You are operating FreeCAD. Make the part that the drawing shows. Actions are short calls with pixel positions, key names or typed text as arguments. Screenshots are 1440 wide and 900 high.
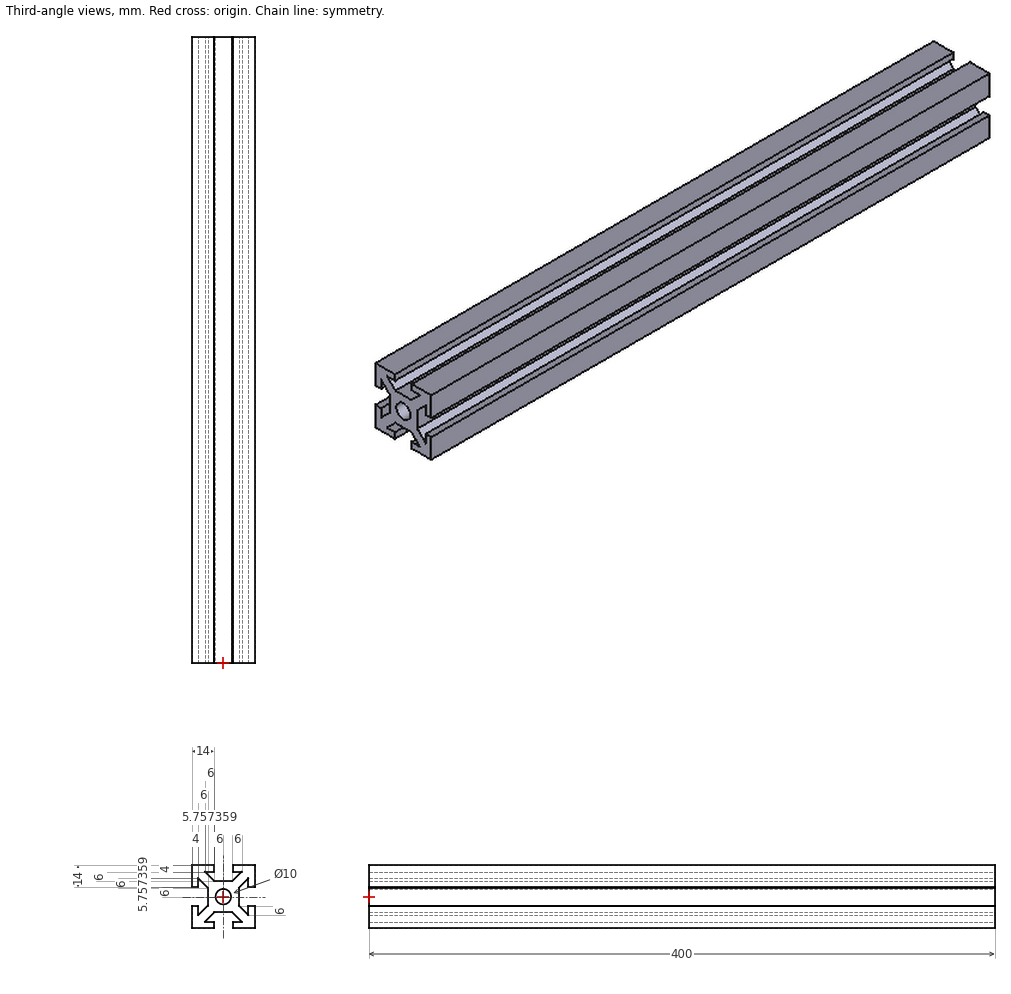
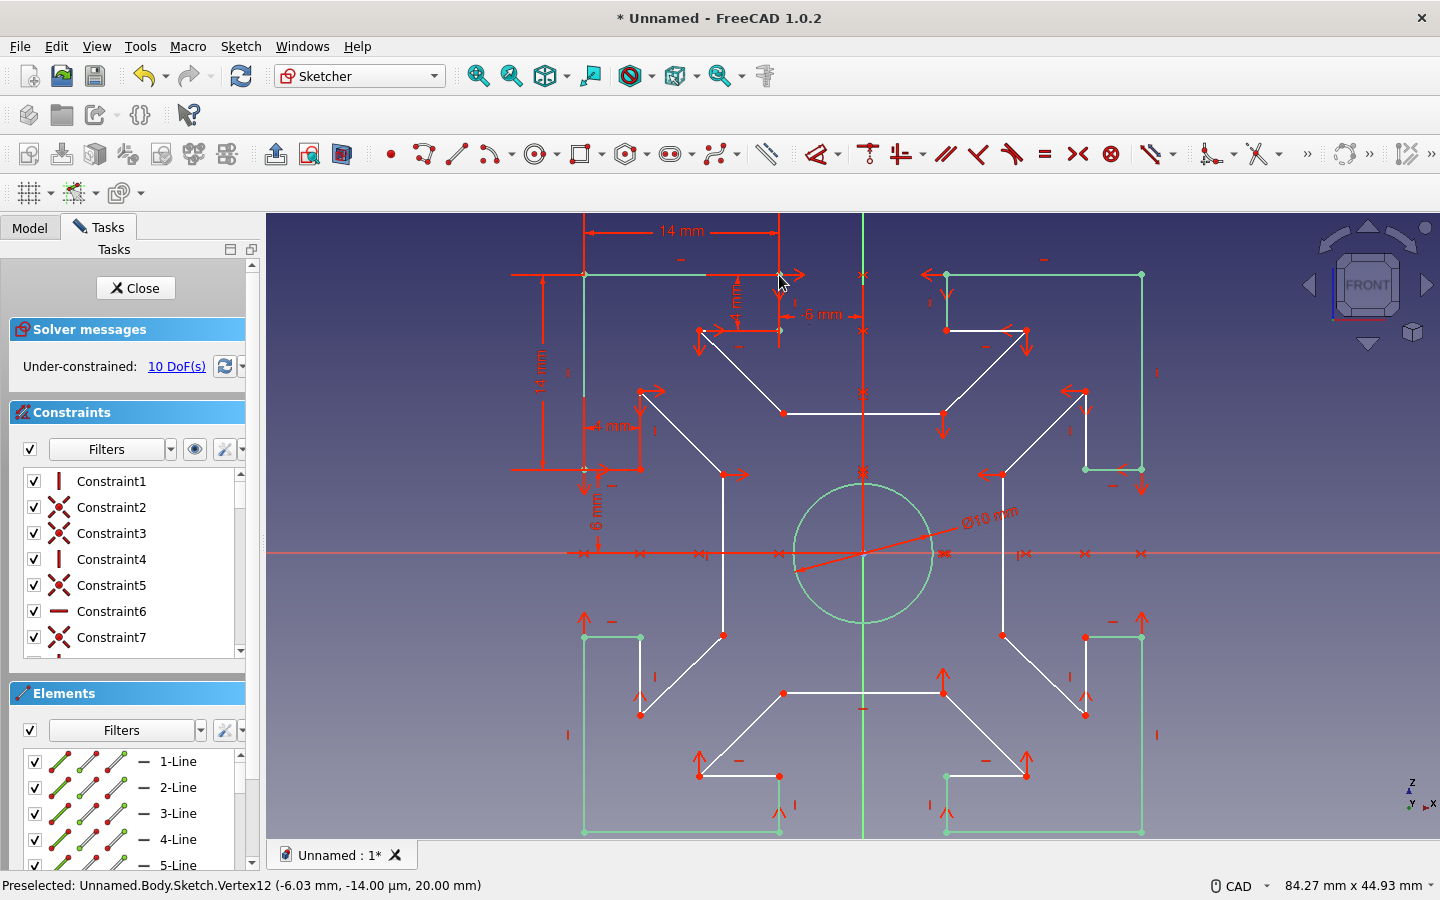
click(698, 450)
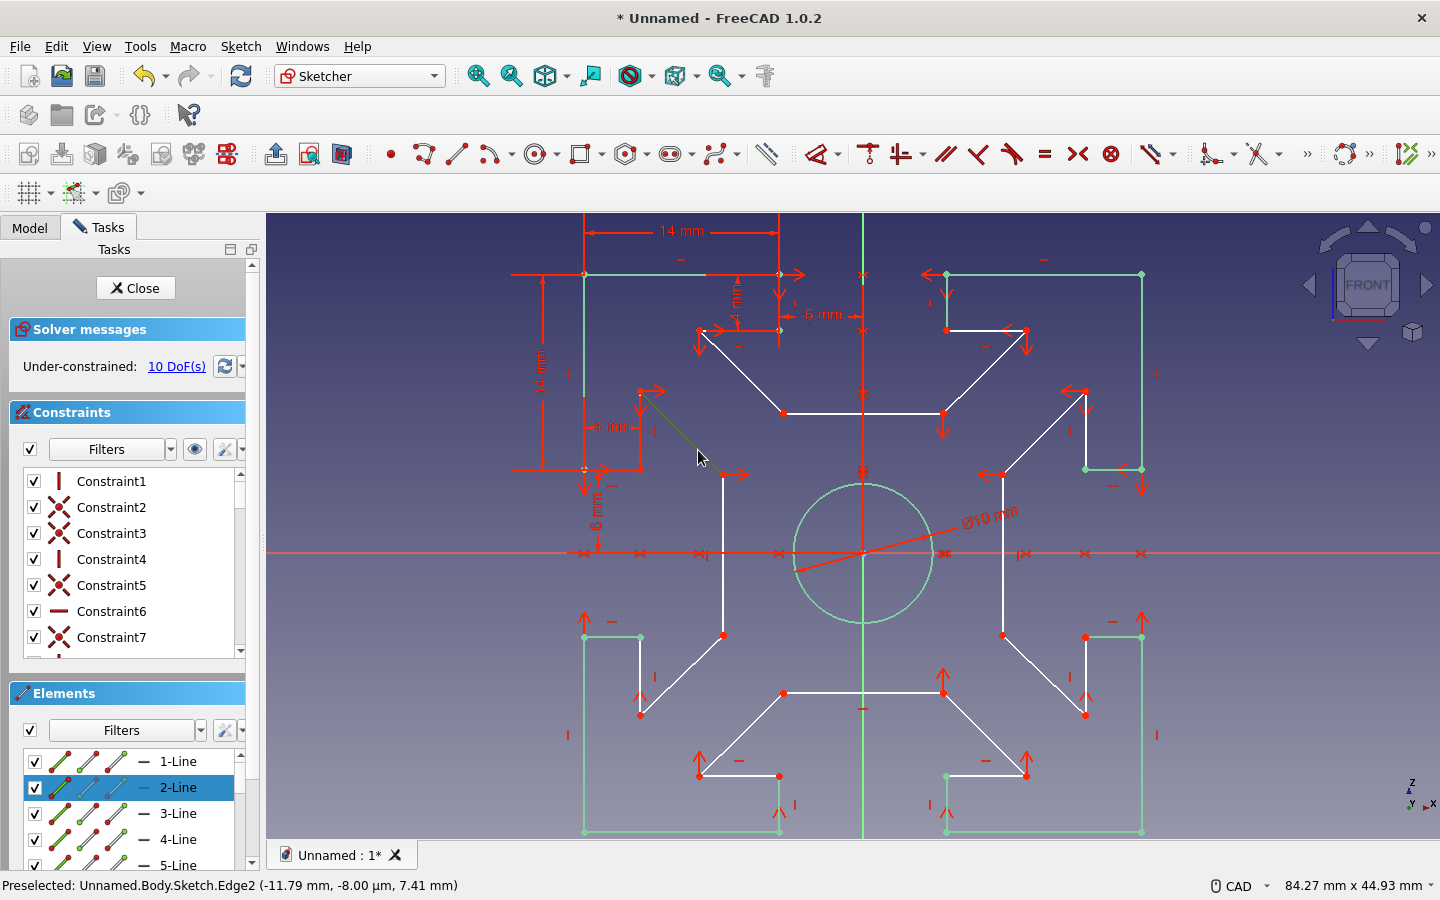
click(838, 154)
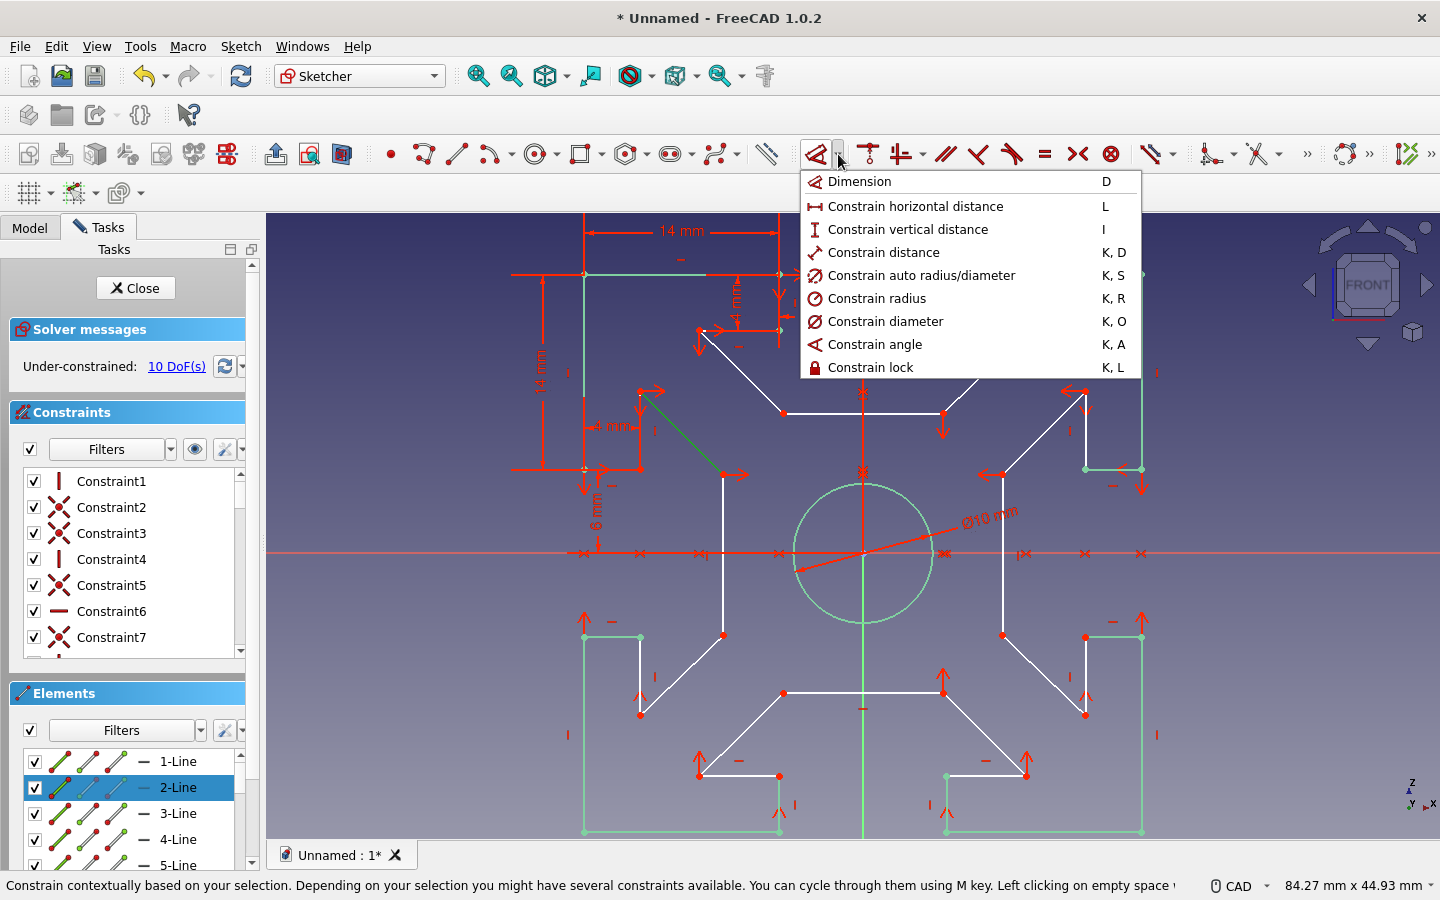
click(971, 206)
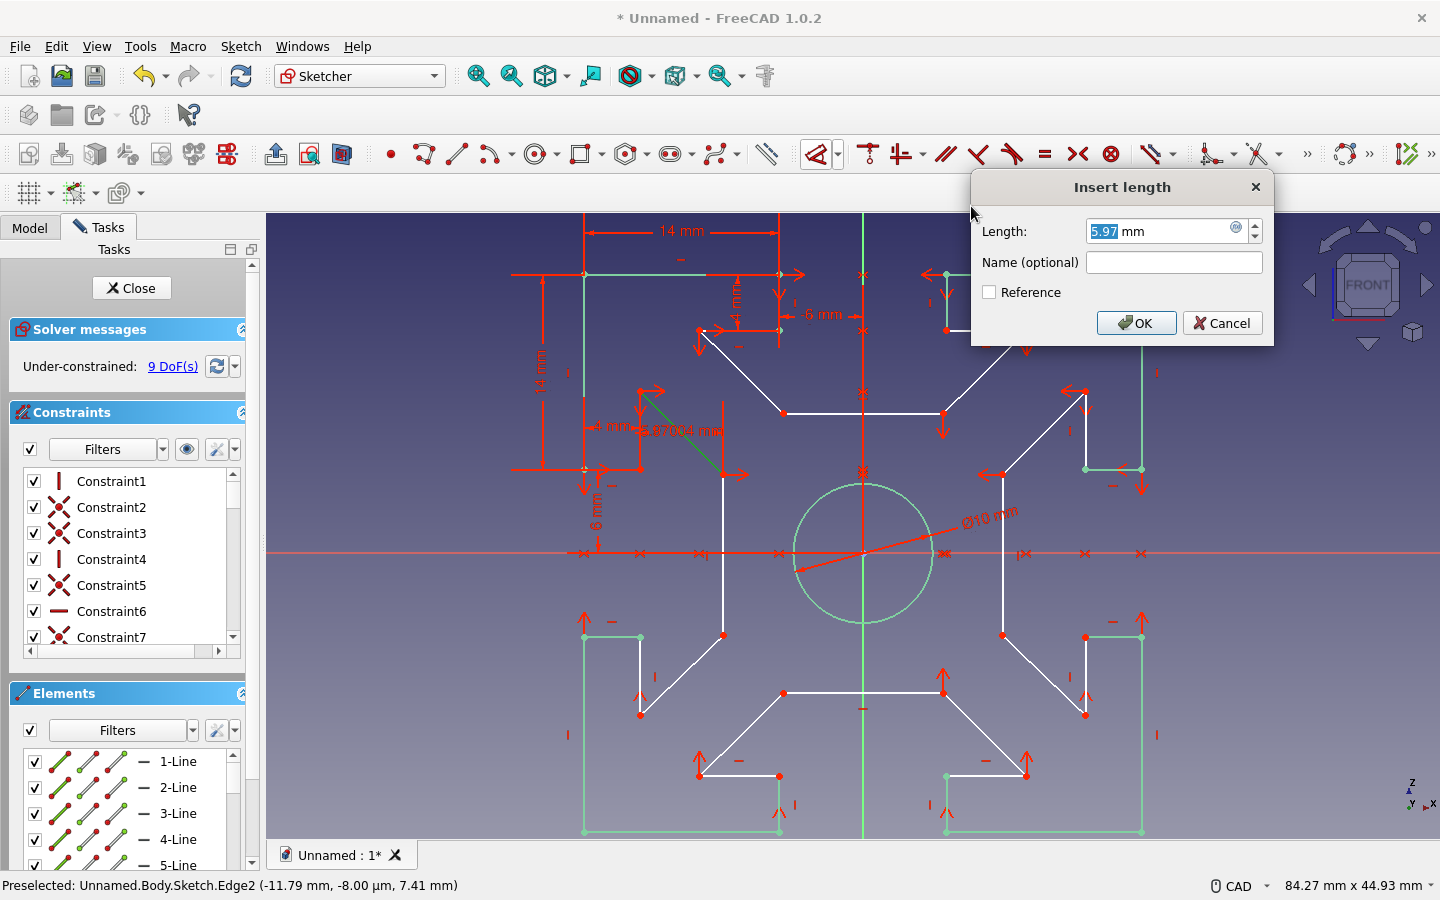
text(6)
key(Return)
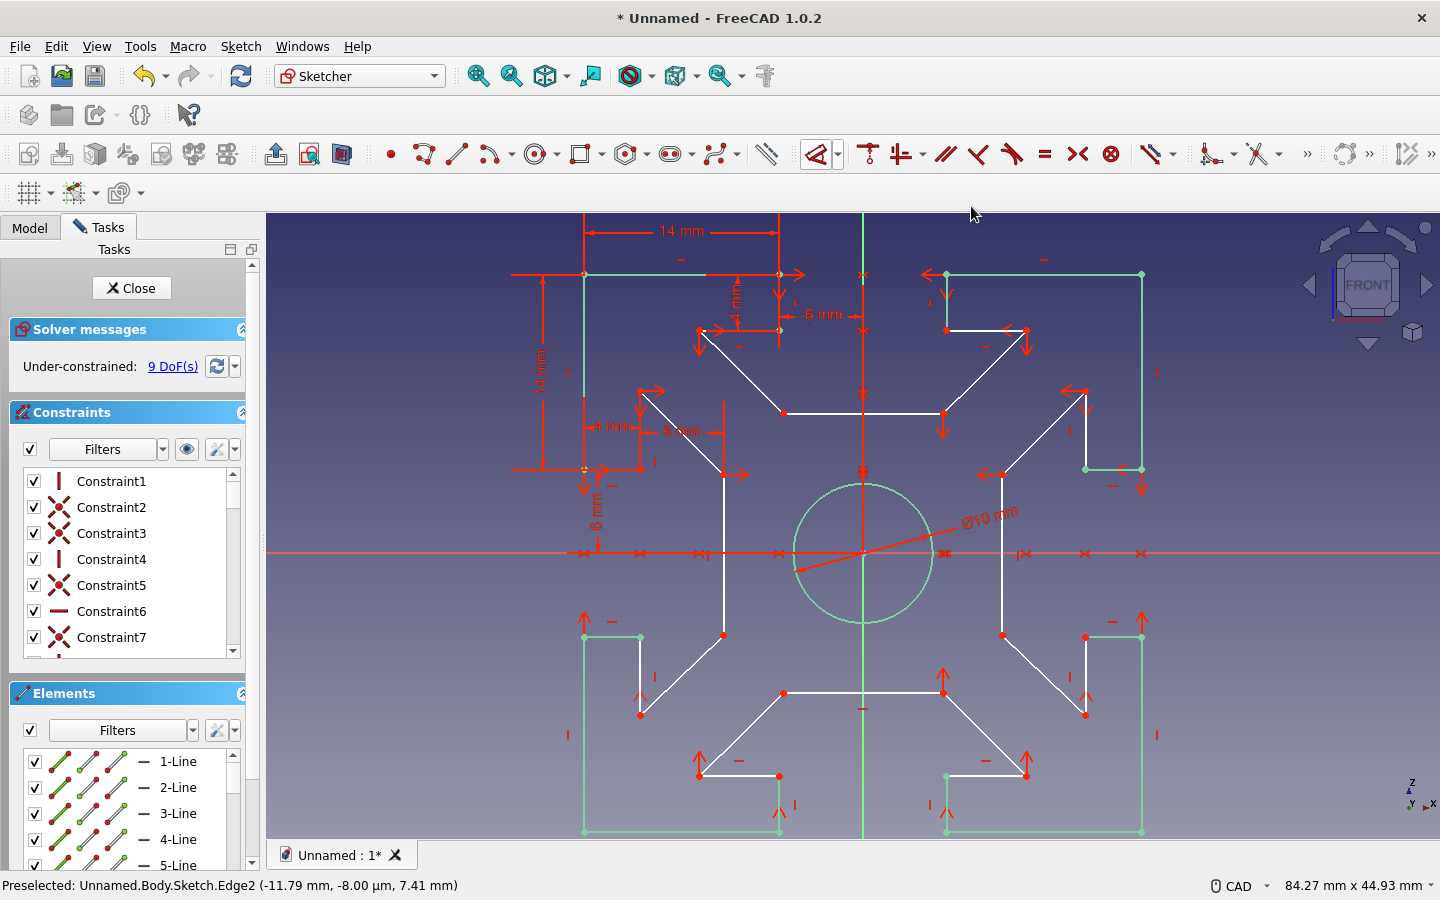
click(699, 450)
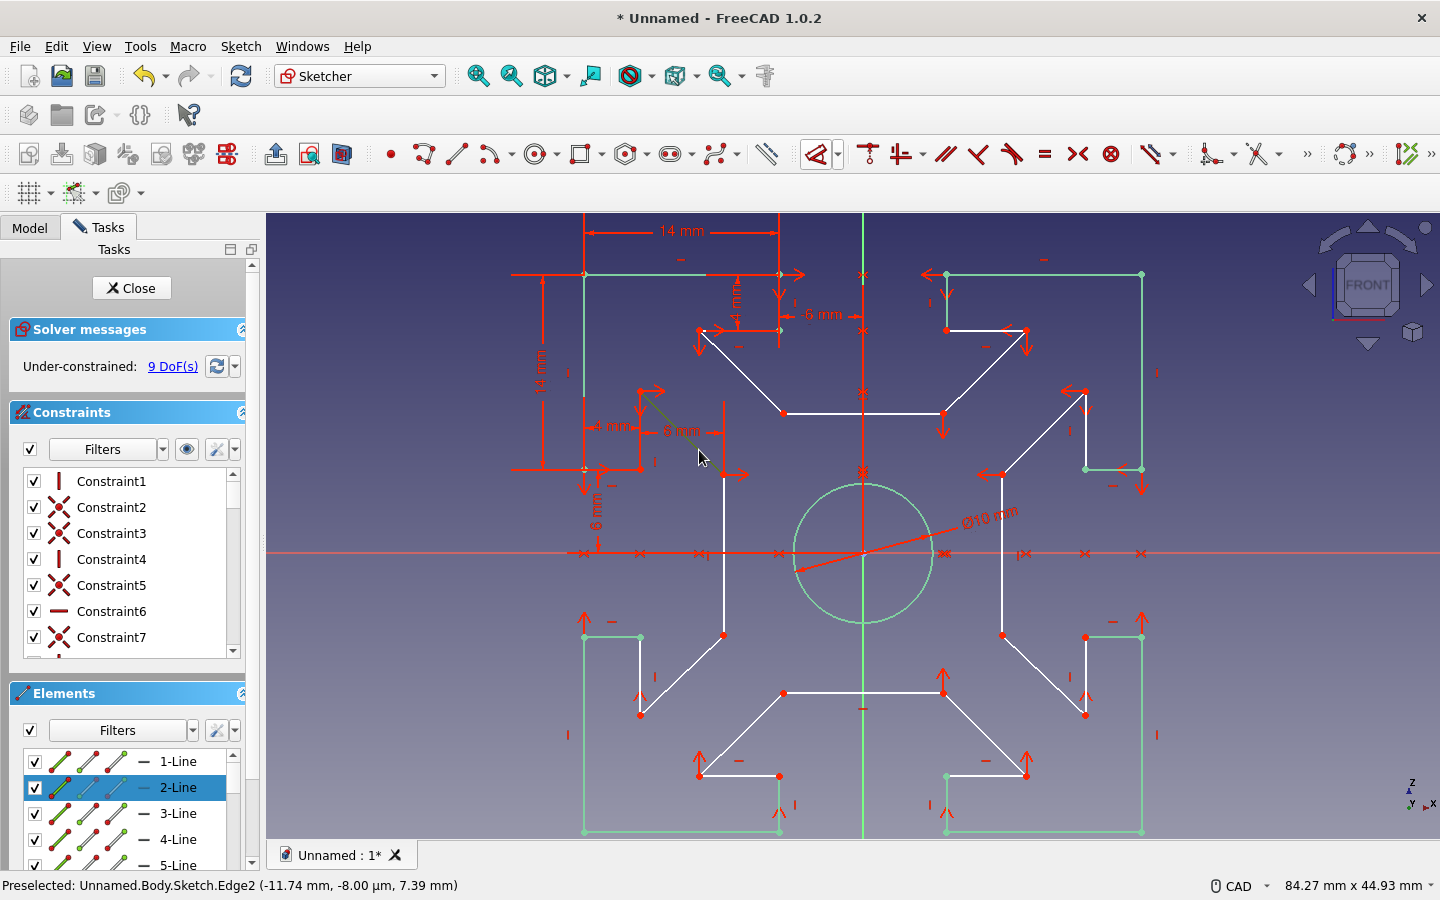
key(i)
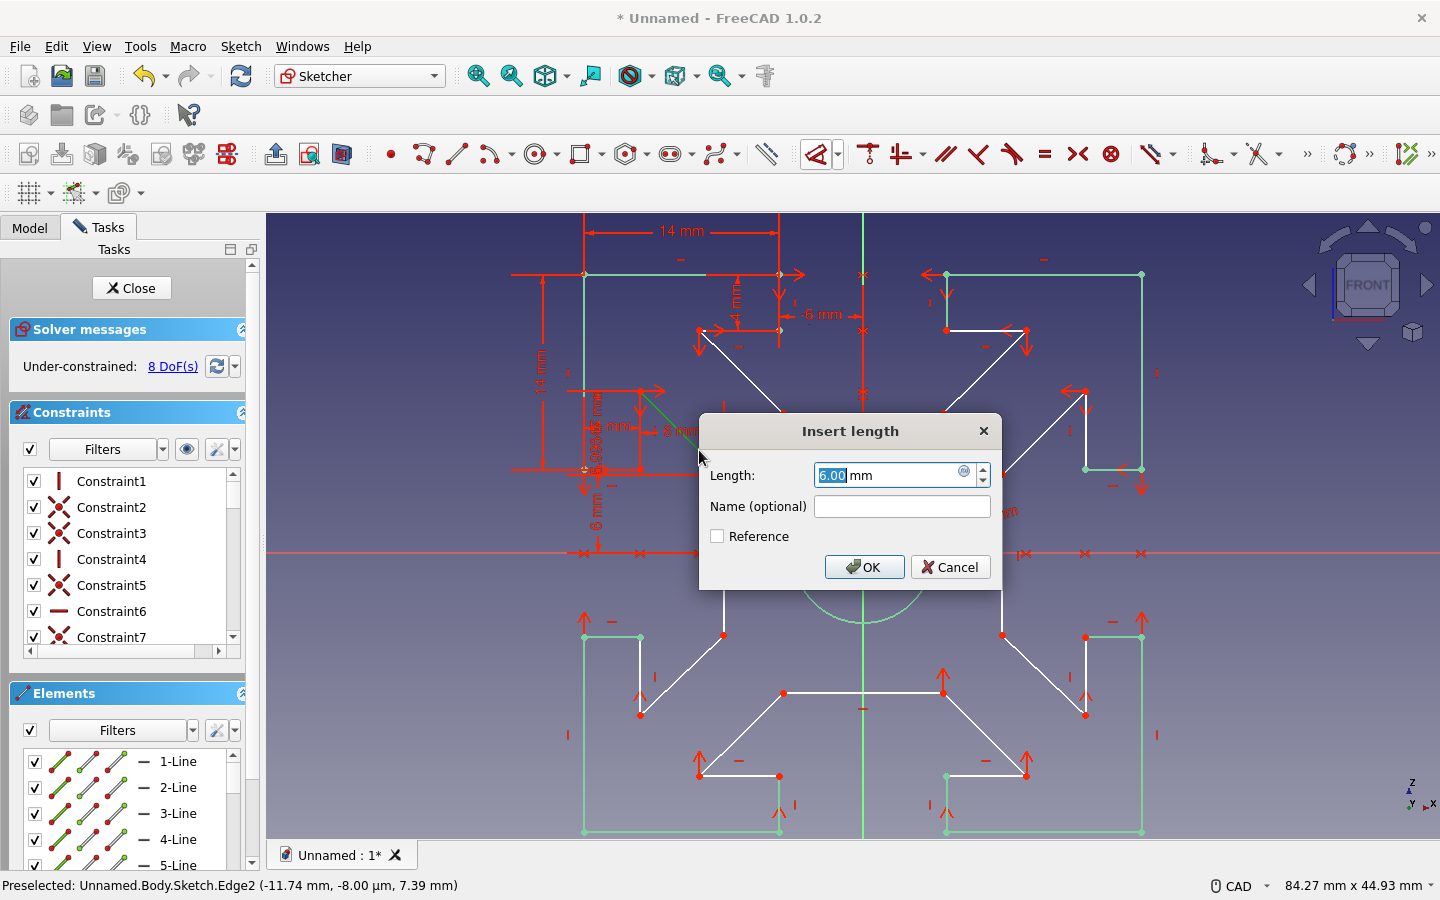
text(6)
key(Return)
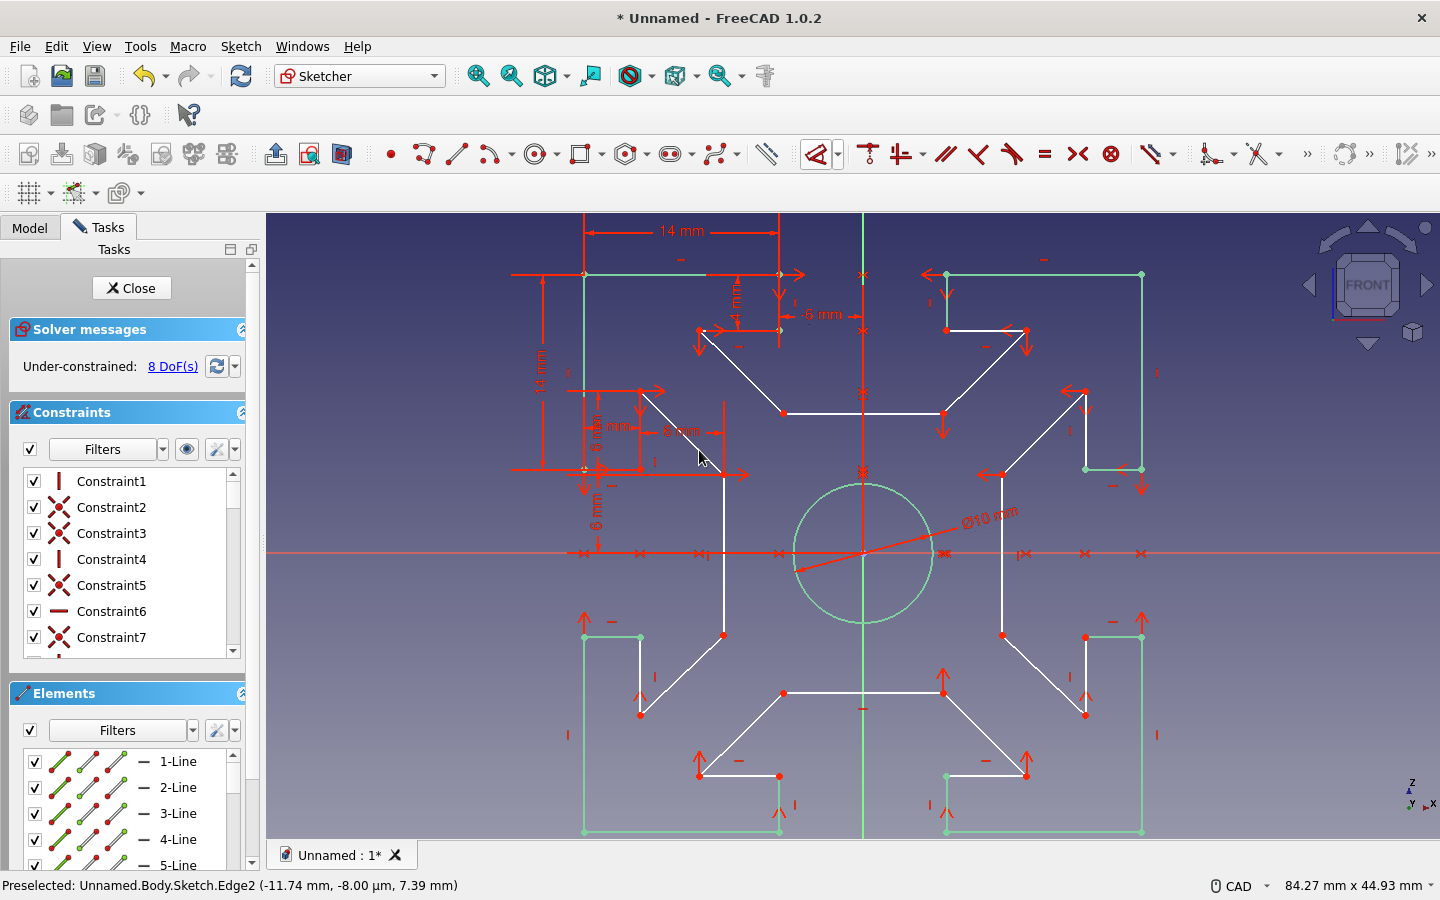
click(725, 356)